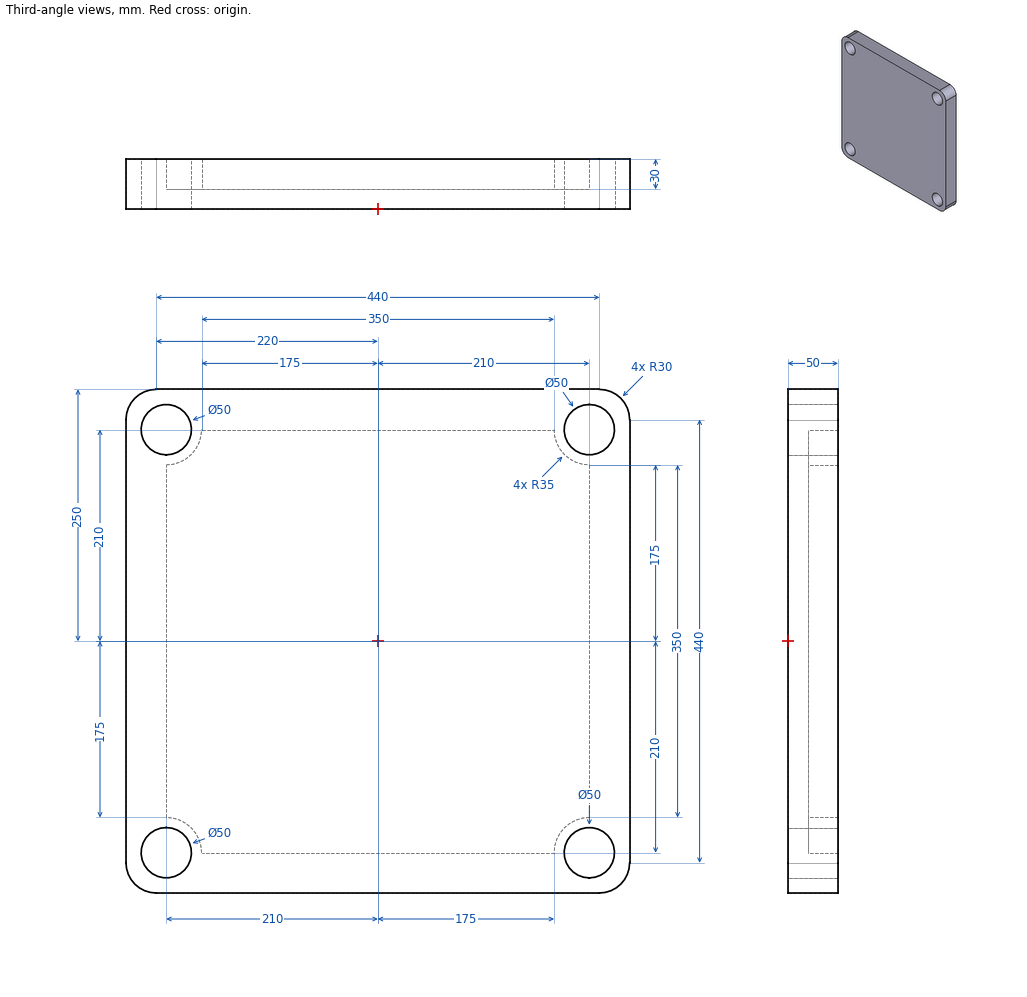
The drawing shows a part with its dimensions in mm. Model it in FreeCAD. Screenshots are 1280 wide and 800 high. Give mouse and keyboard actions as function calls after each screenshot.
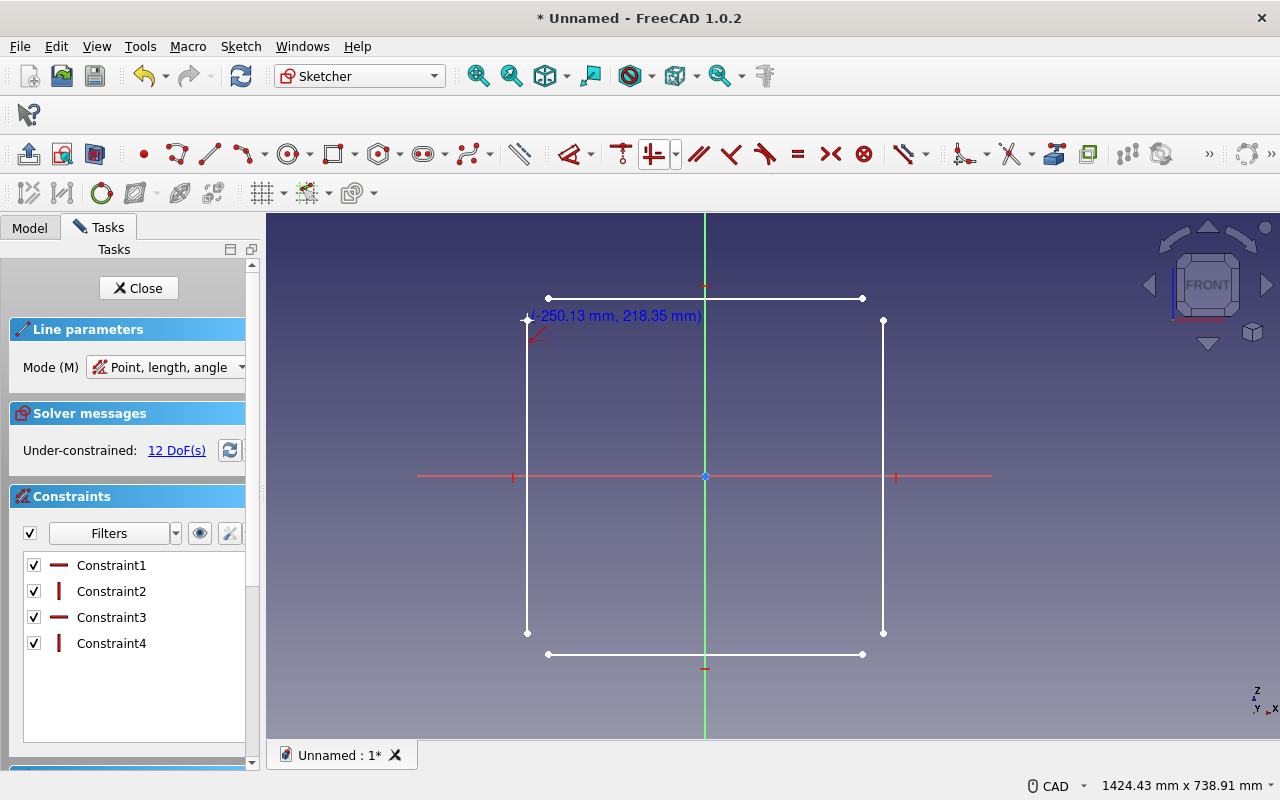
click(242, 154)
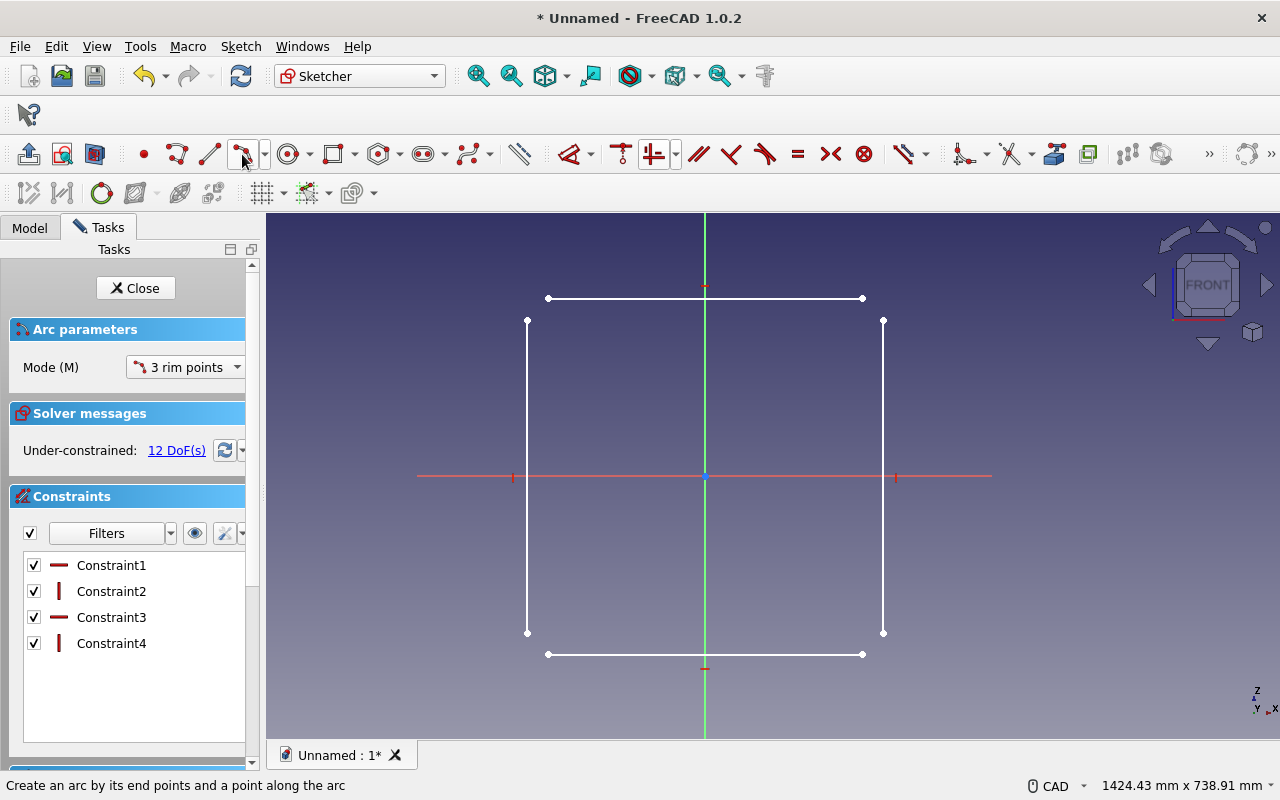
click(862, 299)
click(883, 321)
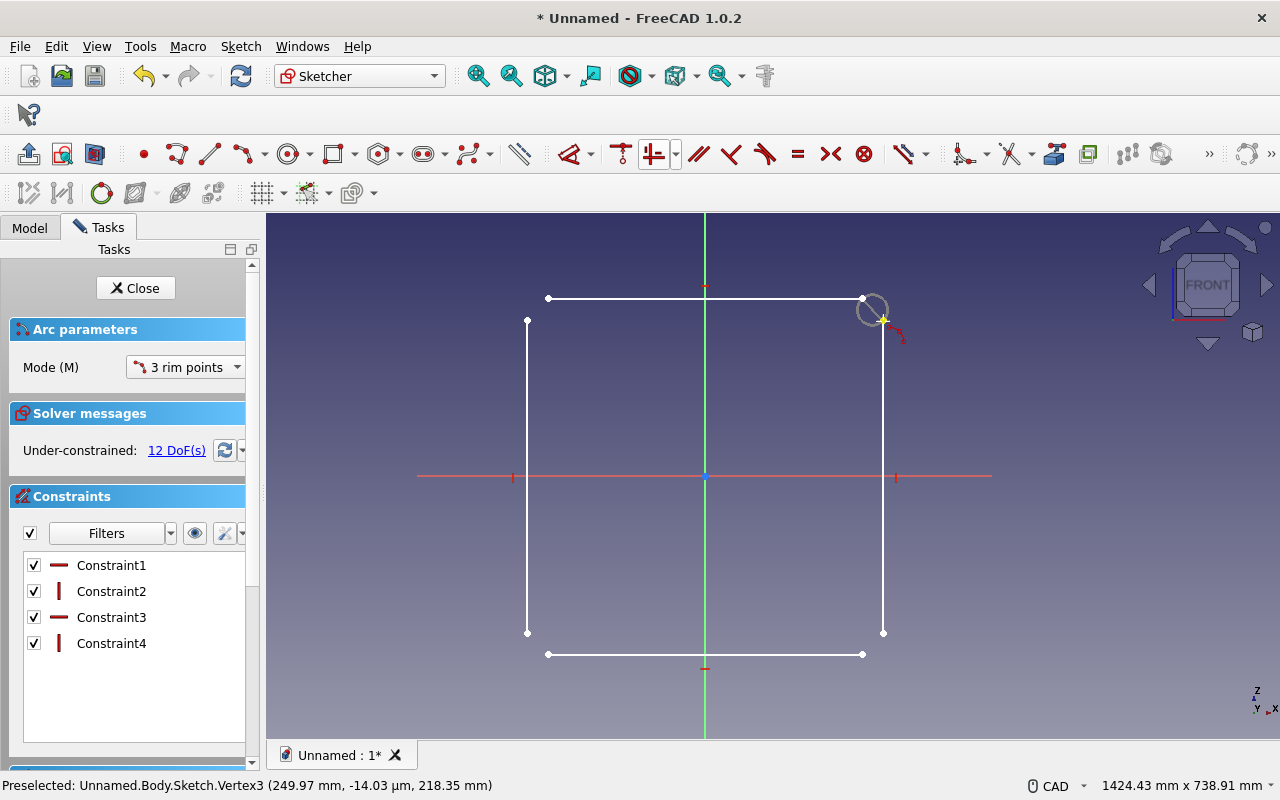
scroll(877, 305, up, 5)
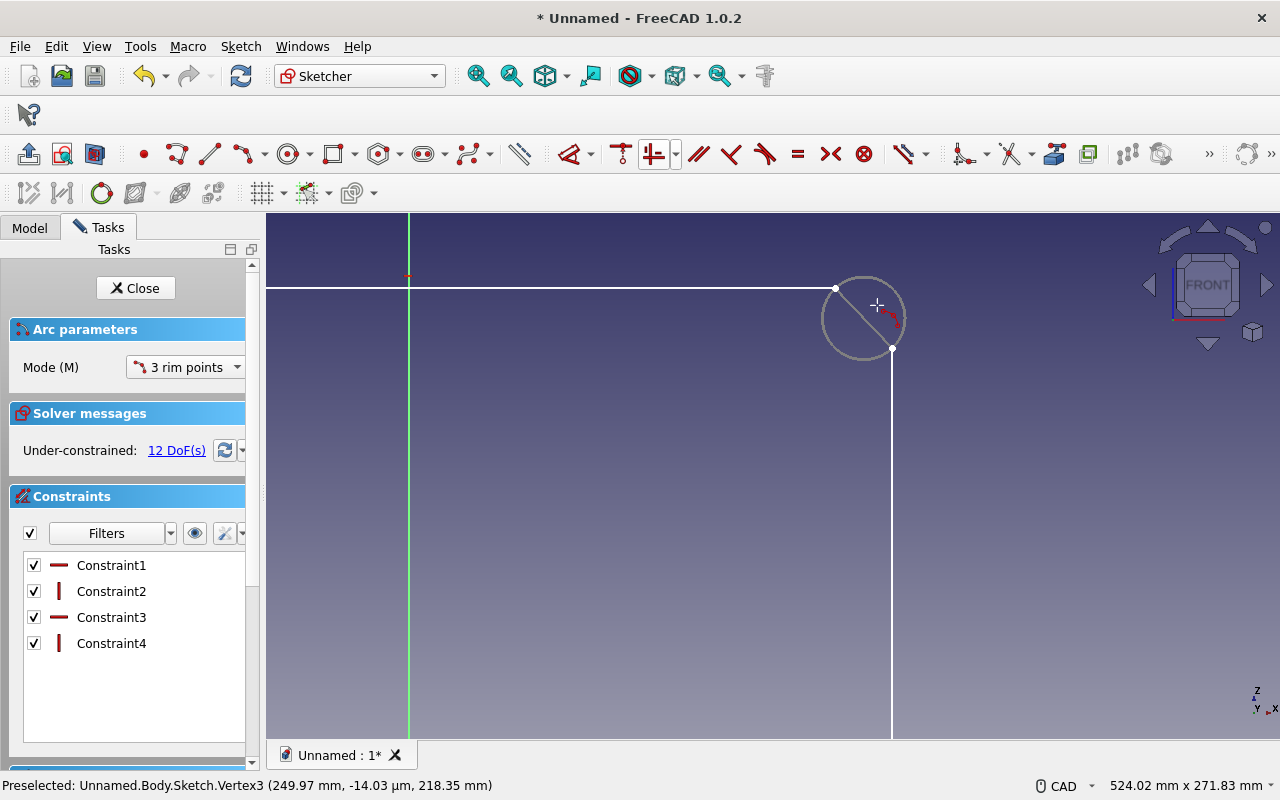
click(875, 304)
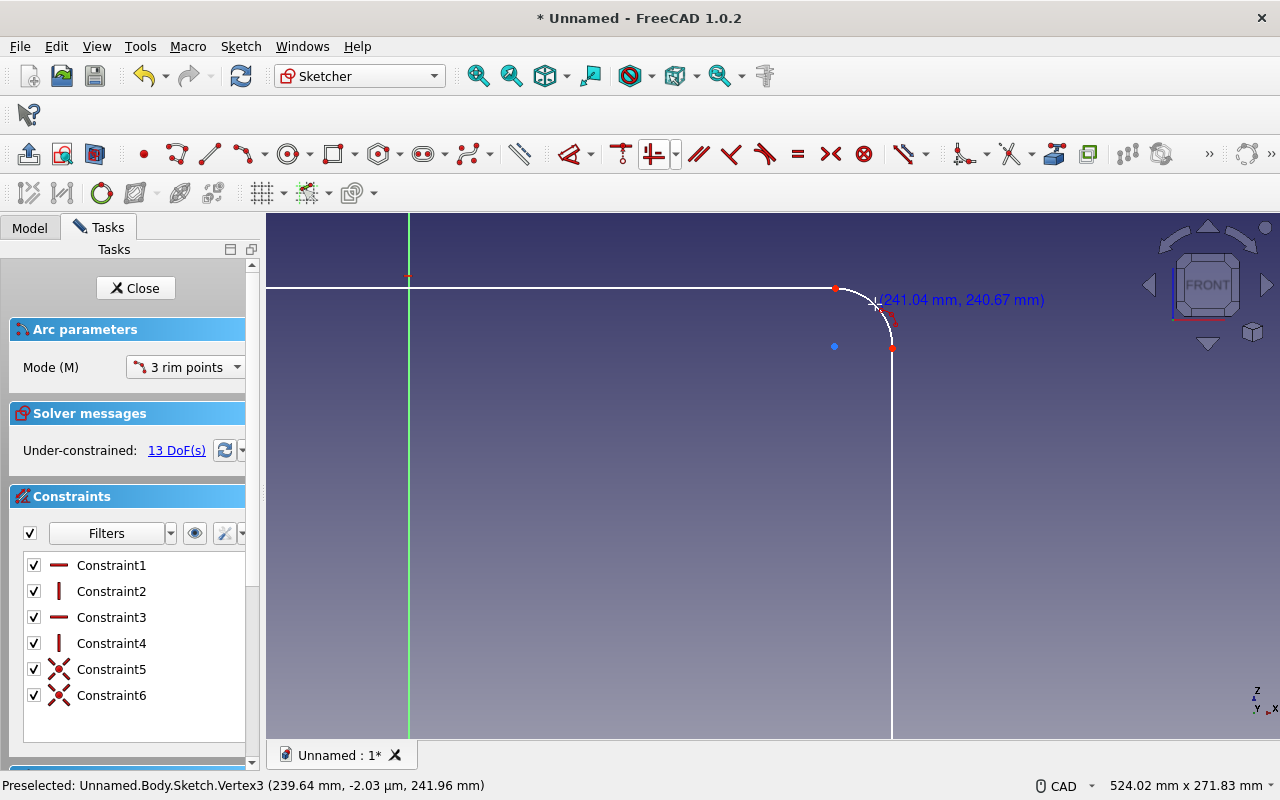
scroll(877, 304, down, 5)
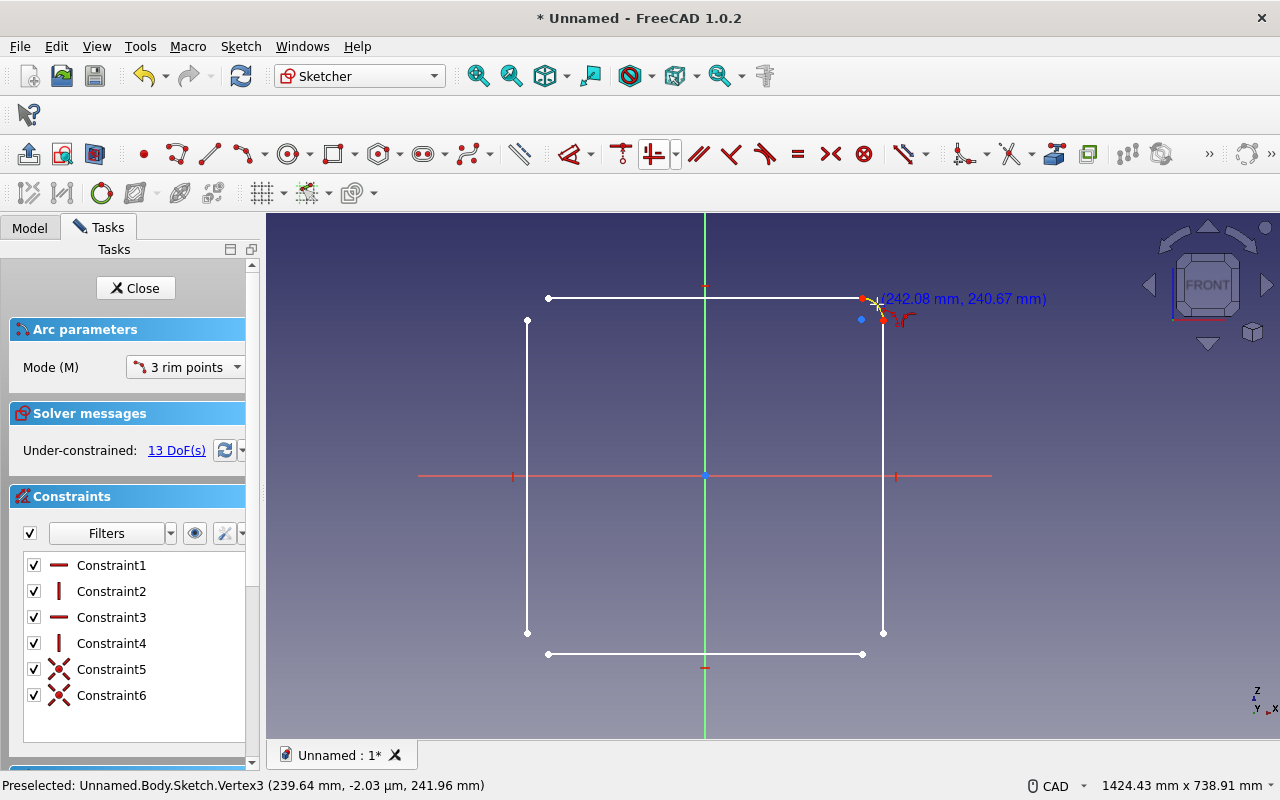
click(883, 633)
click(862, 654)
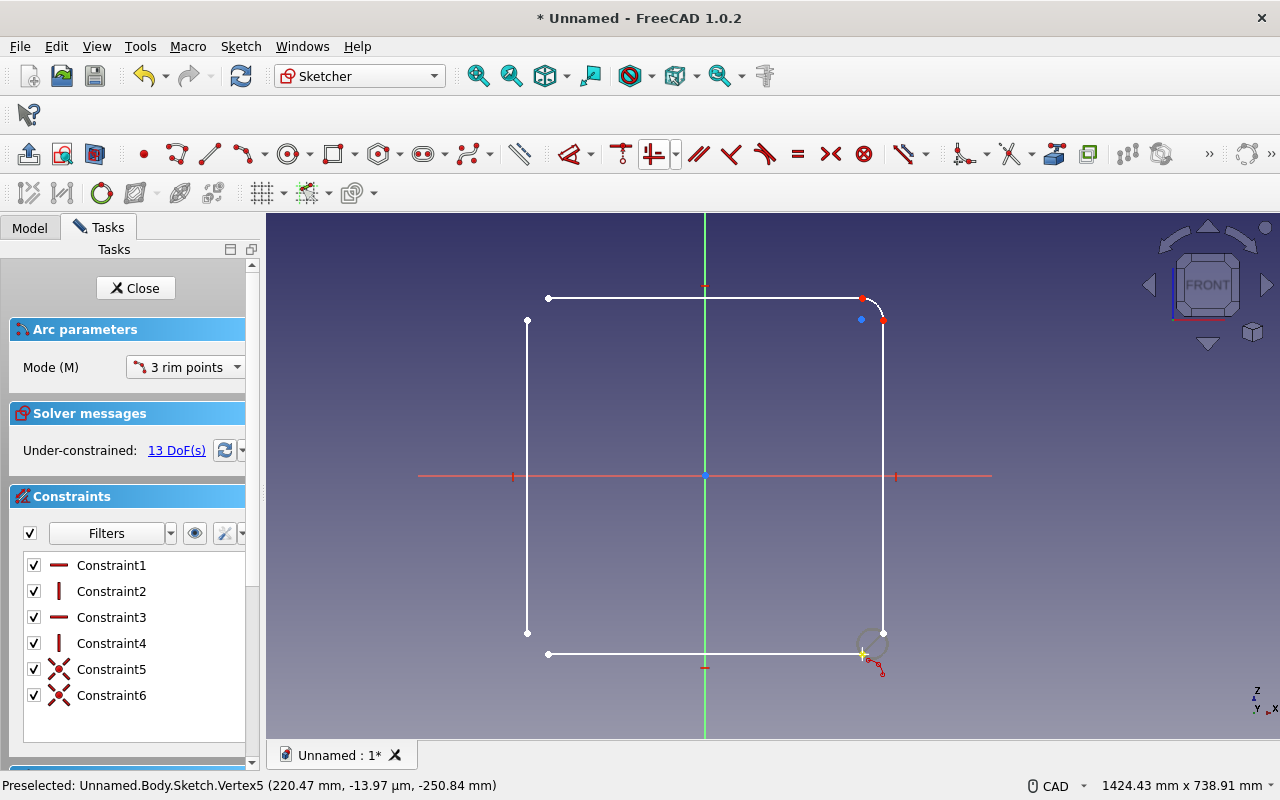
scroll(877, 648, up, 5)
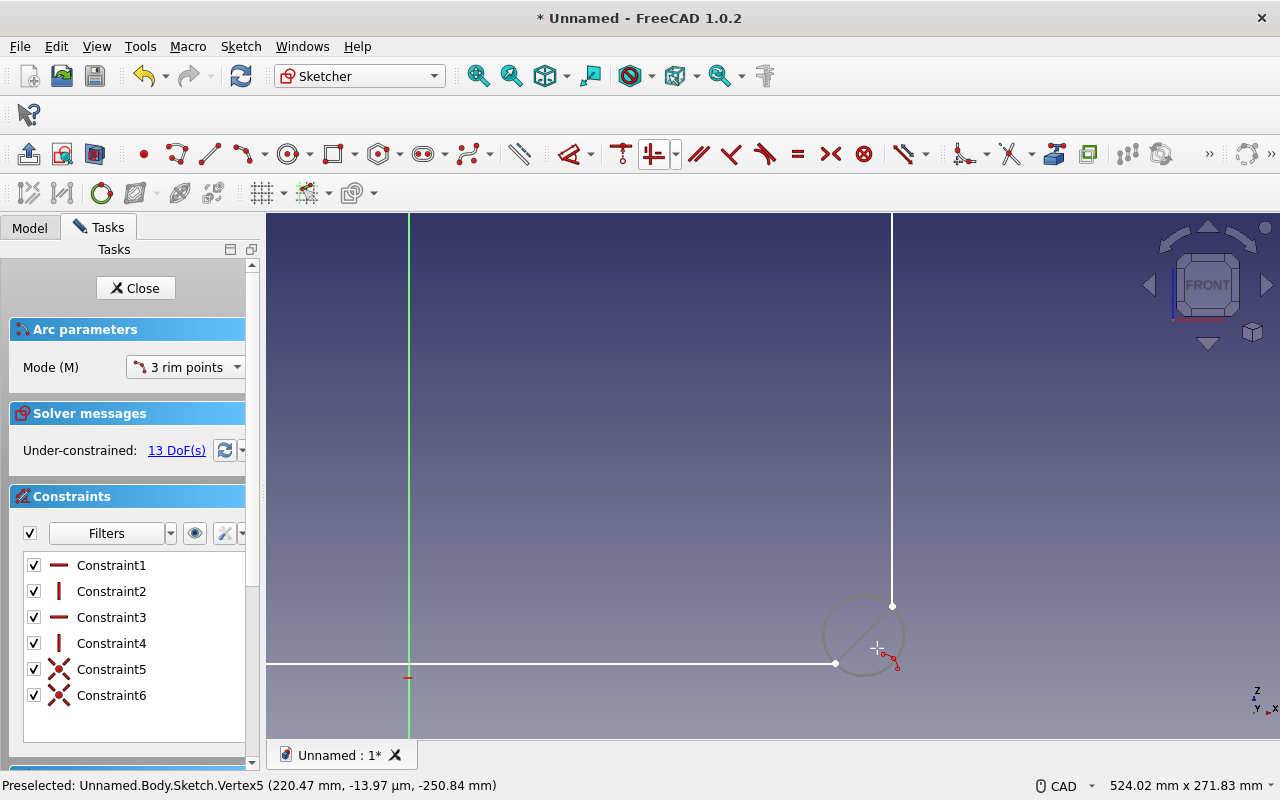
click(875, 645)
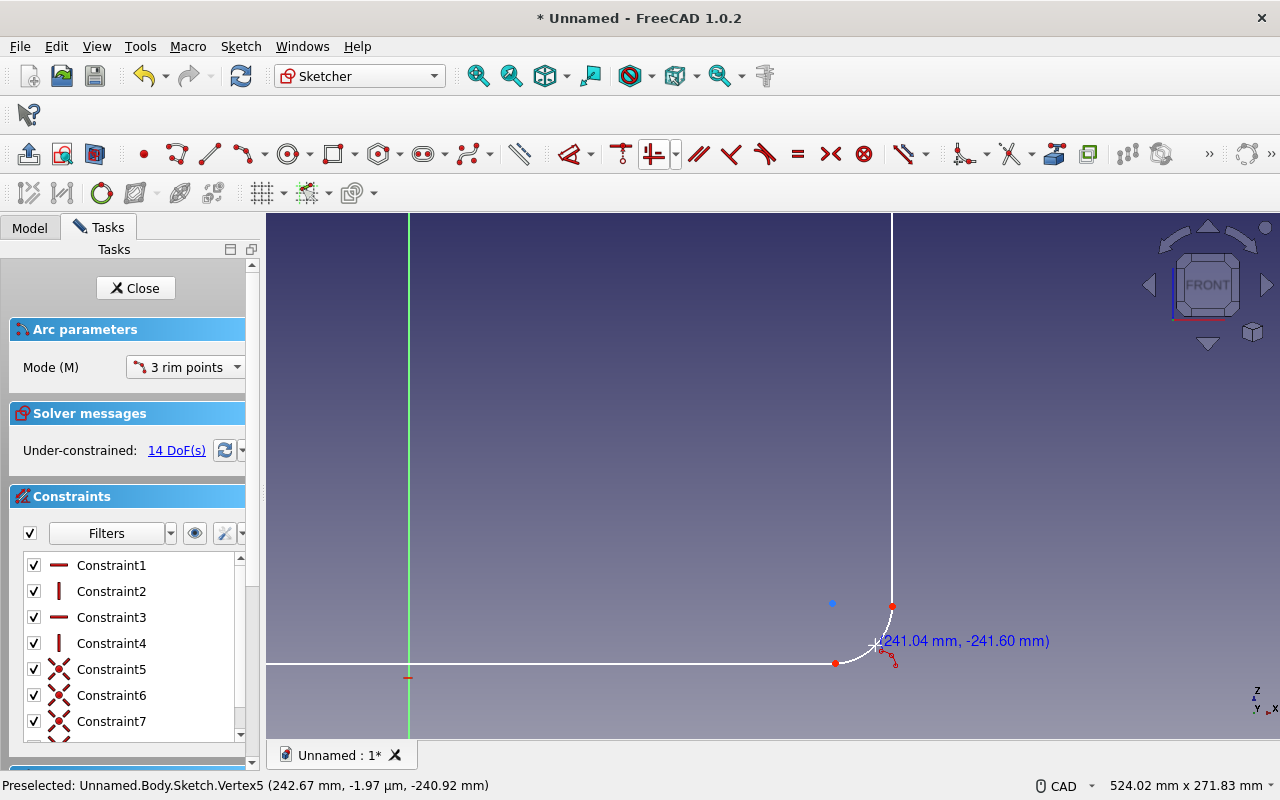
scroll(877, 649, down, 5)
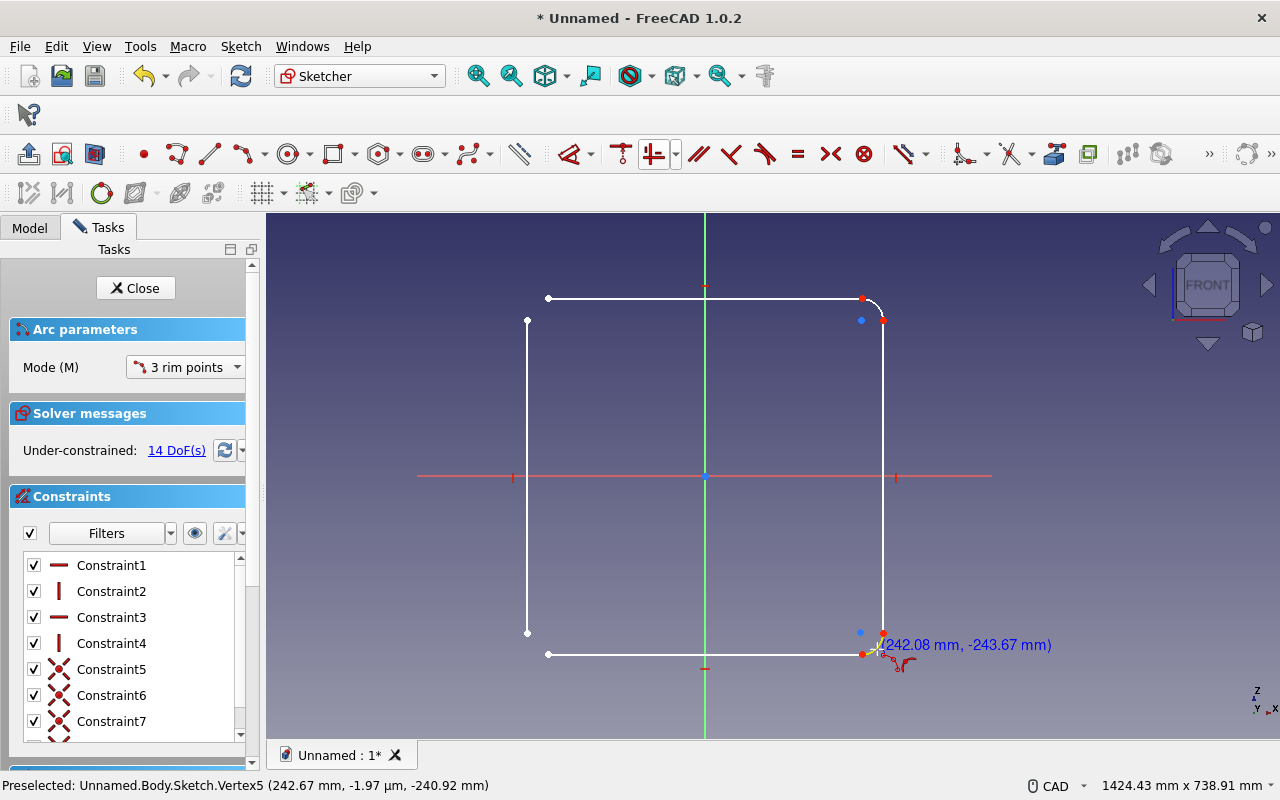
click(548, 655)
click(527, 634)